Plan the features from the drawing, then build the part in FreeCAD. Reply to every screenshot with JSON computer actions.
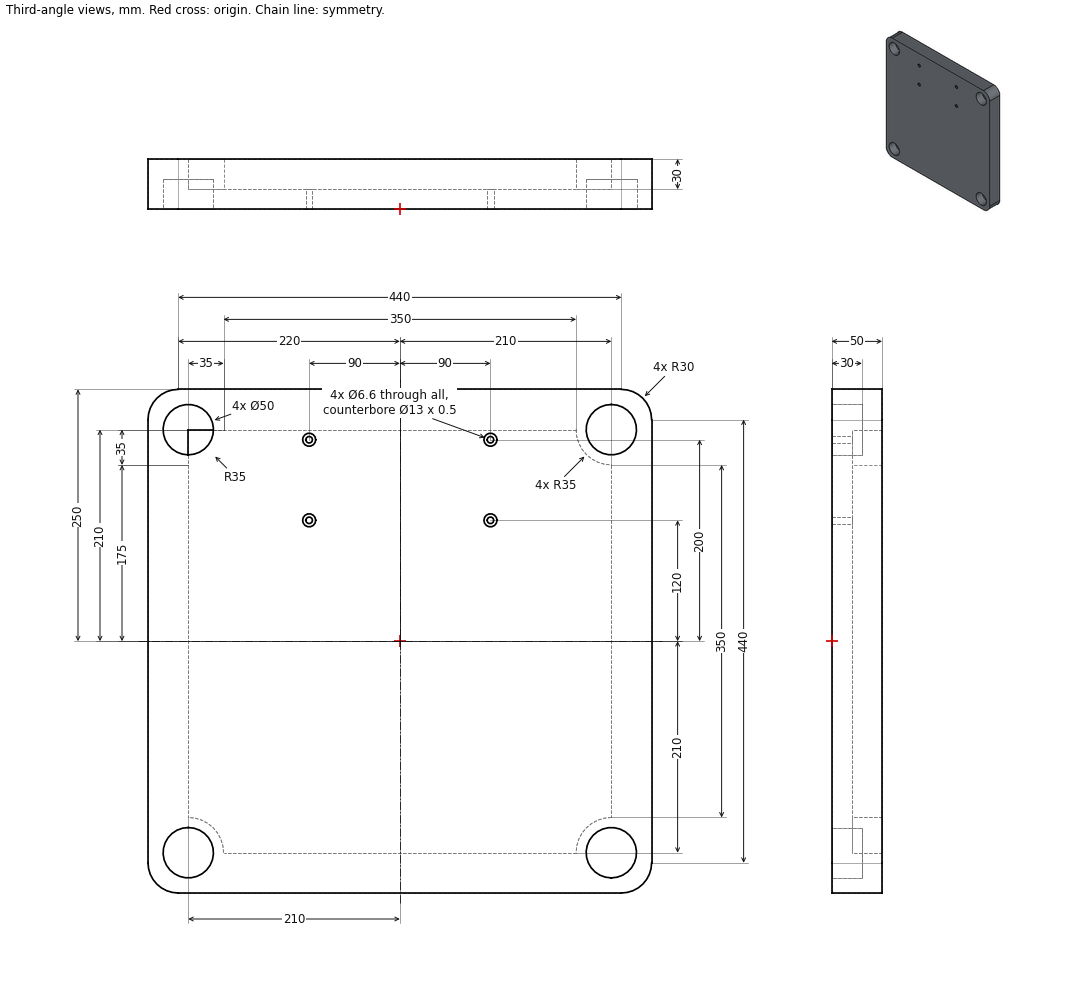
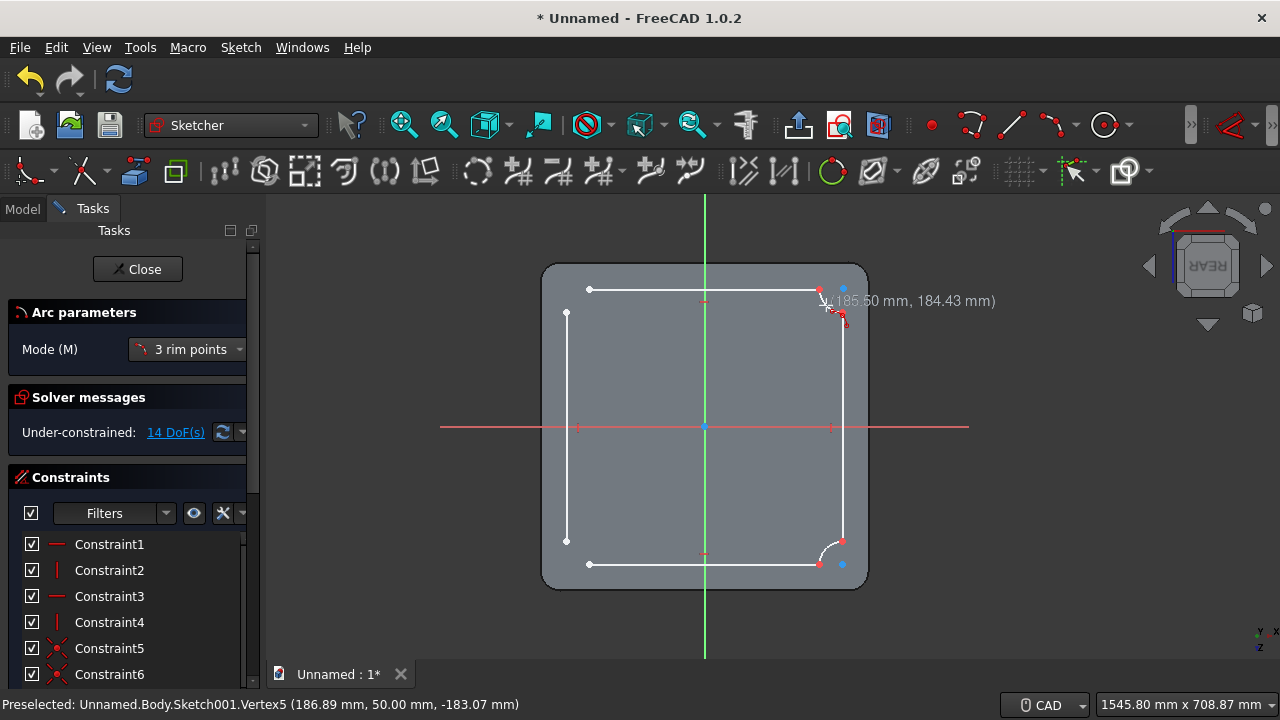
{"action": "left_click", "coordinate": [590, 290]}
{"action": "left_click", "coordinate": [567, 313]}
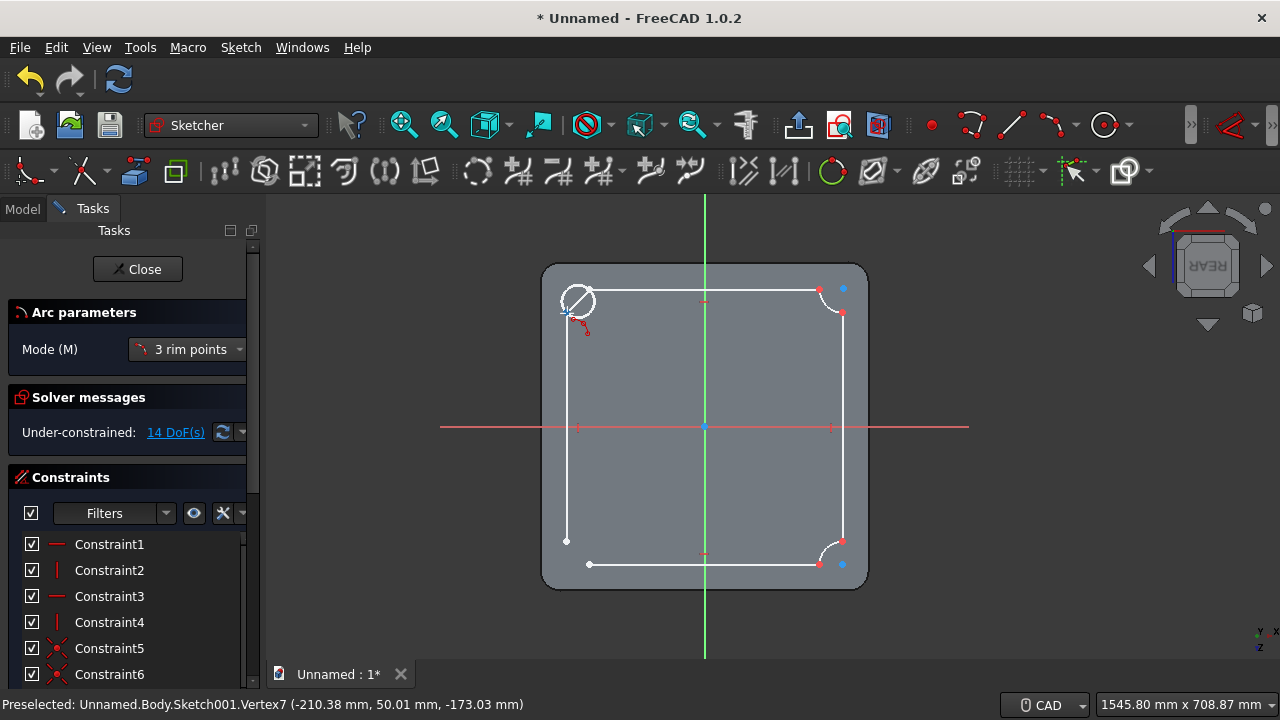
{"action": "scroll", "coordinate": [583, 305], "scroll_direction": "up", "scroll_amount": 5}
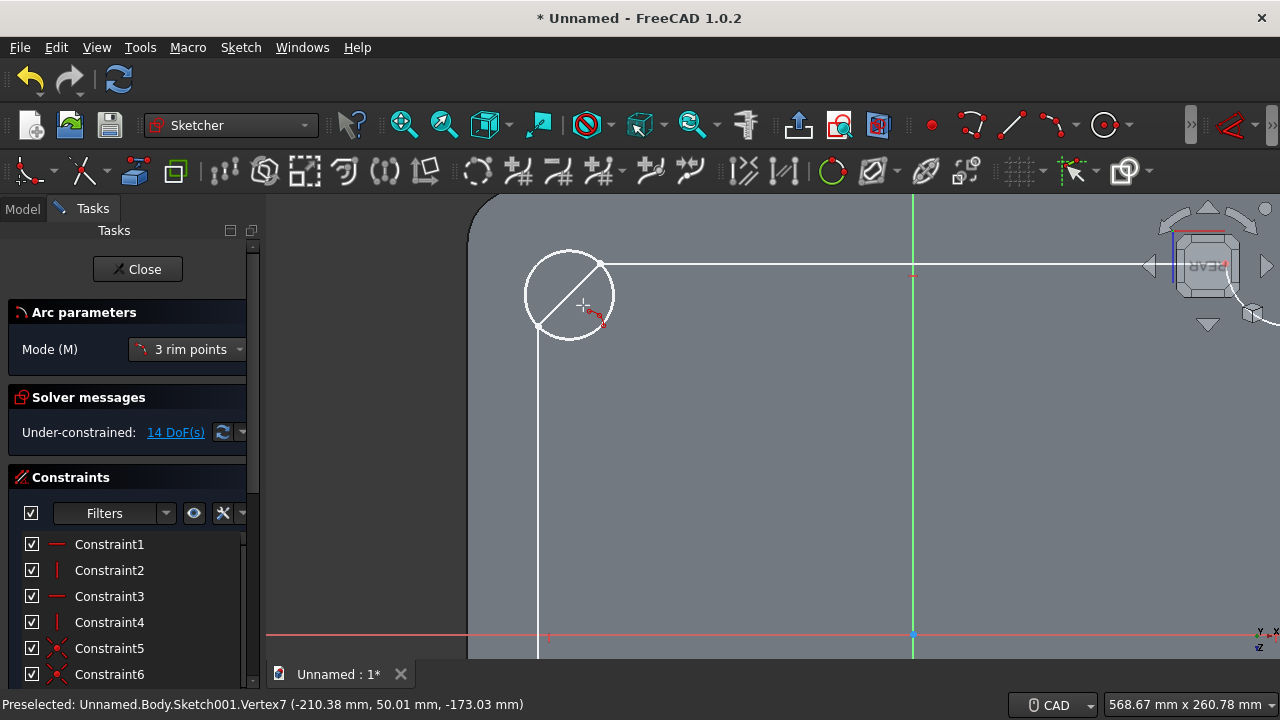
{"action": "left_click", "coordinate": [583, 305]}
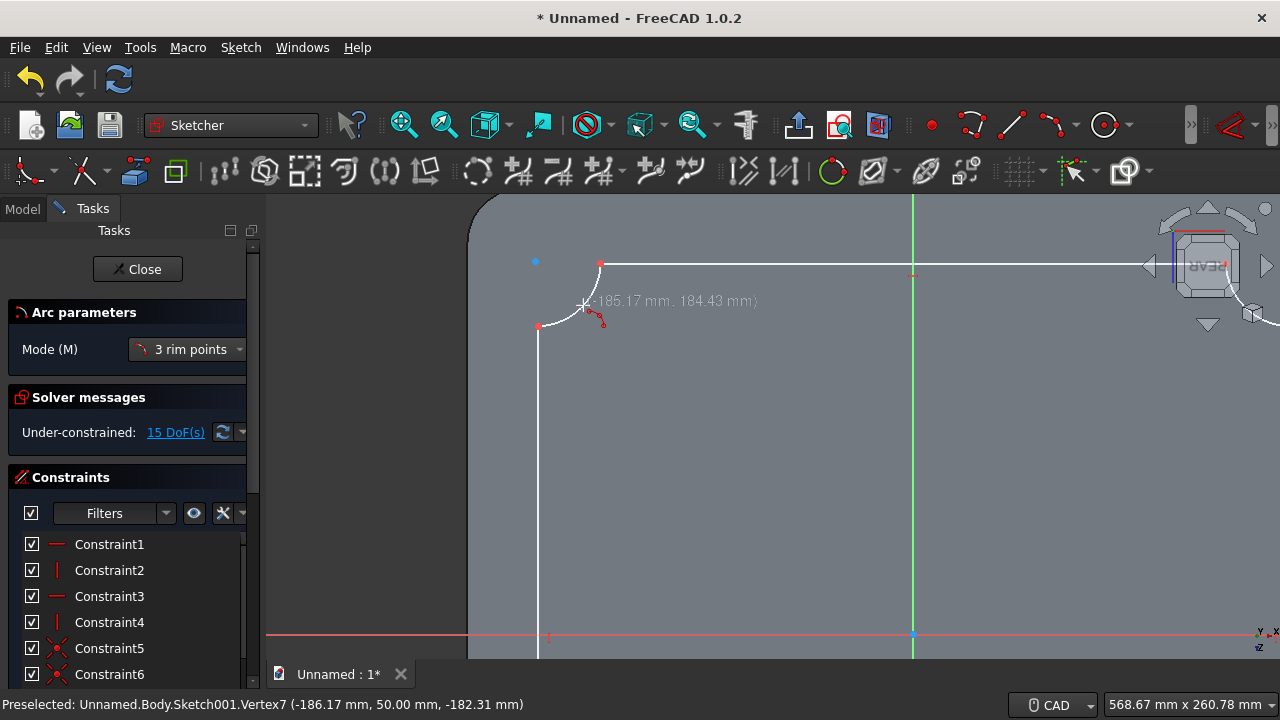
{"action": "scroll", "coordinate": [583, 305], "scroll_direction": "down", "scroll_amount": 5}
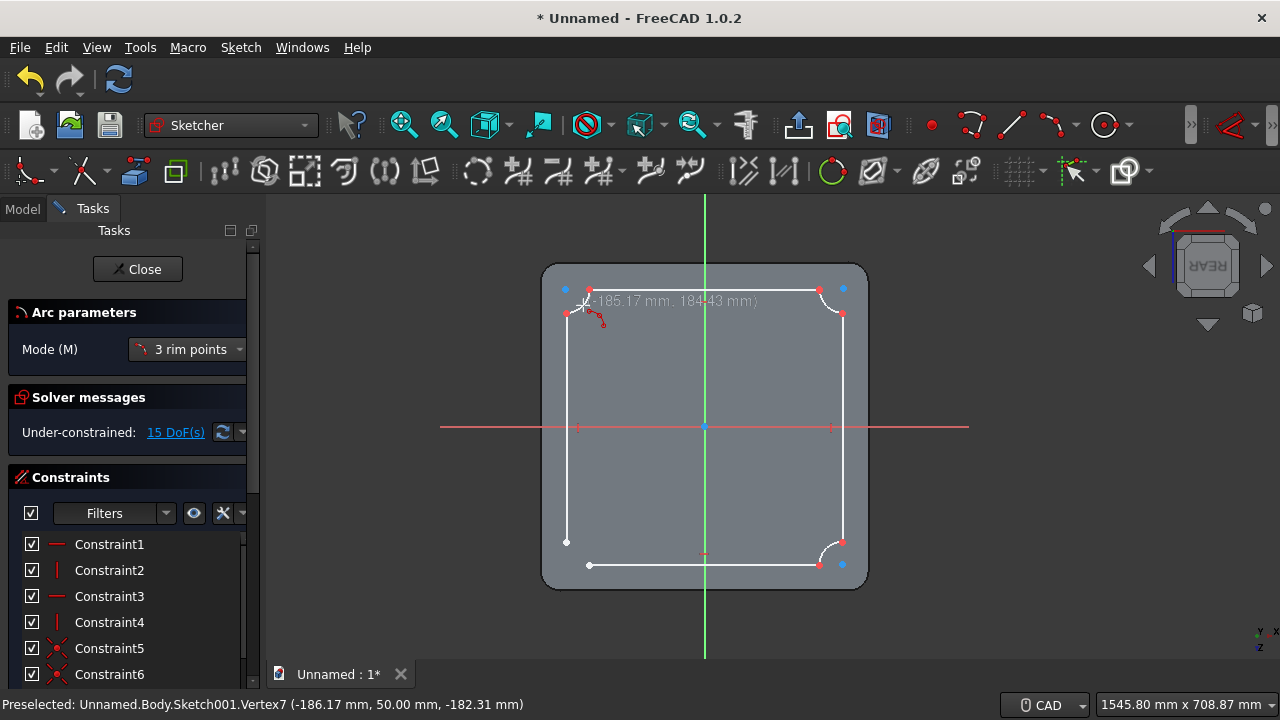
{"action": "left_click", "coordinate": [567, 542]}
{"action": "left_click", "coordinate": [590, 565]}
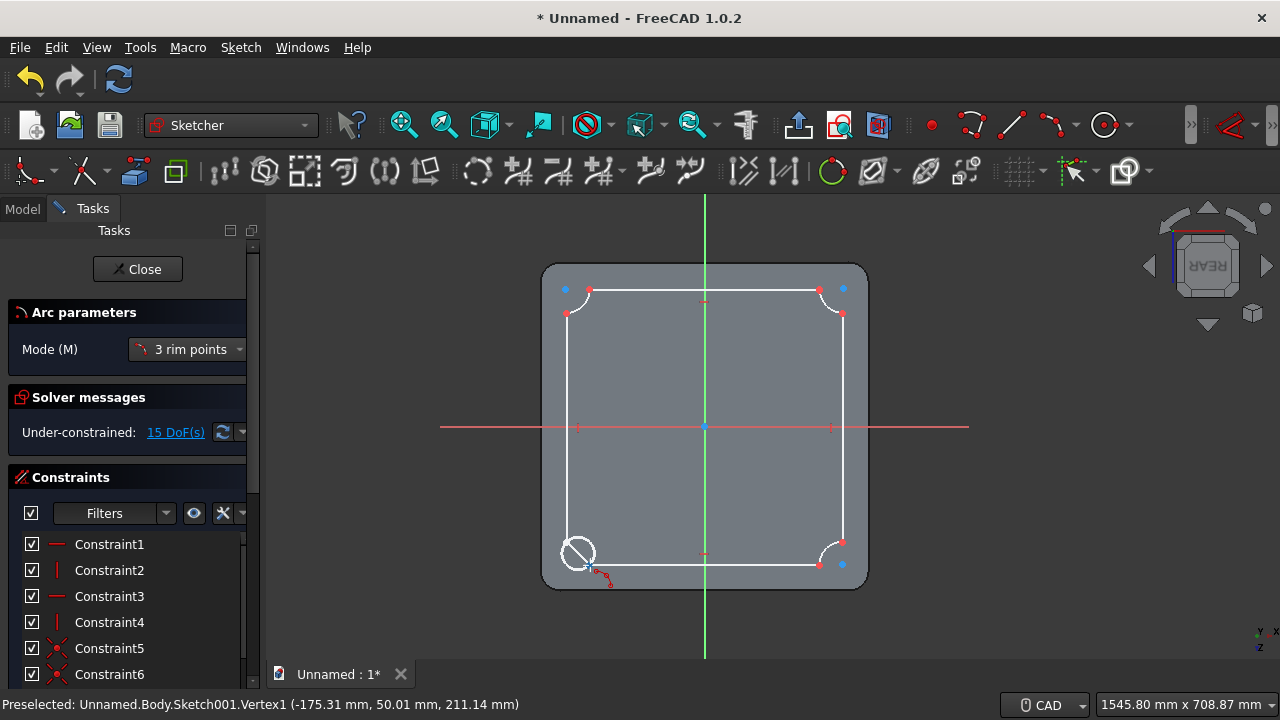
{"action": "scroll", "coordinate": [583, 548], "scroll_direction": "up", "scroll_amount": 5}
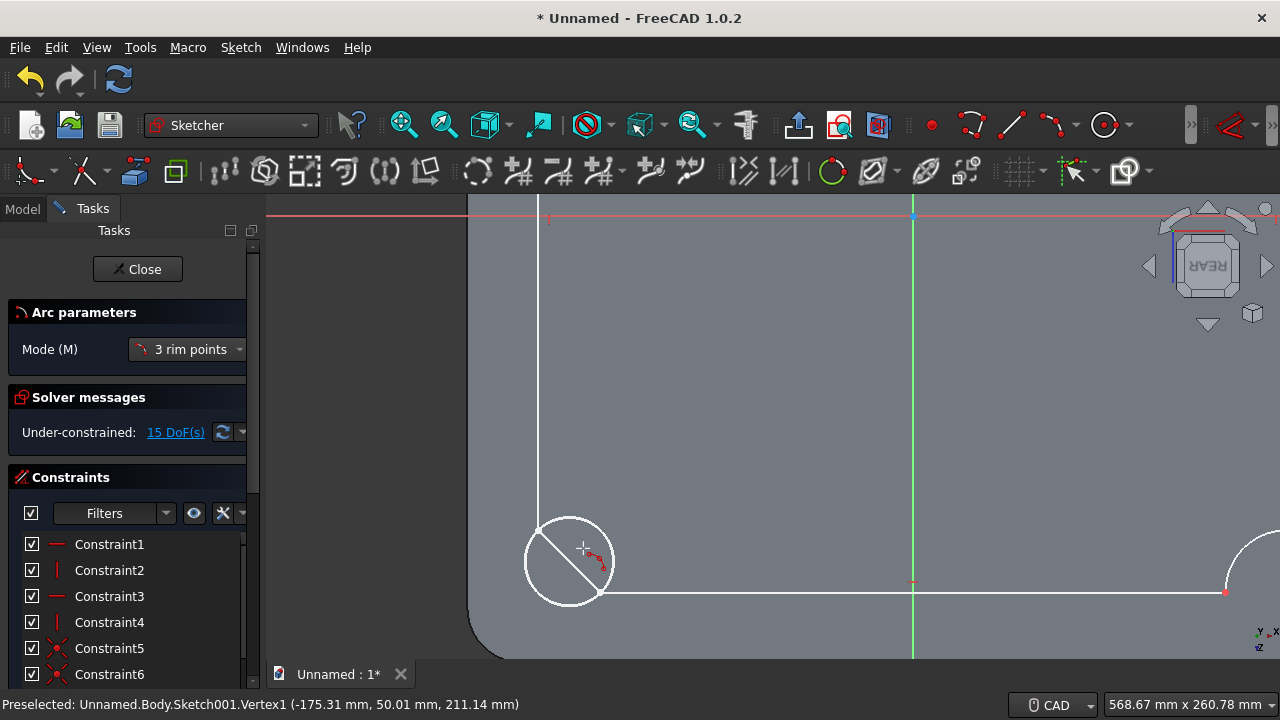
{"action": "left_click", "coordinate": [583, 547]}
{"action": "key", "text": "Escape"}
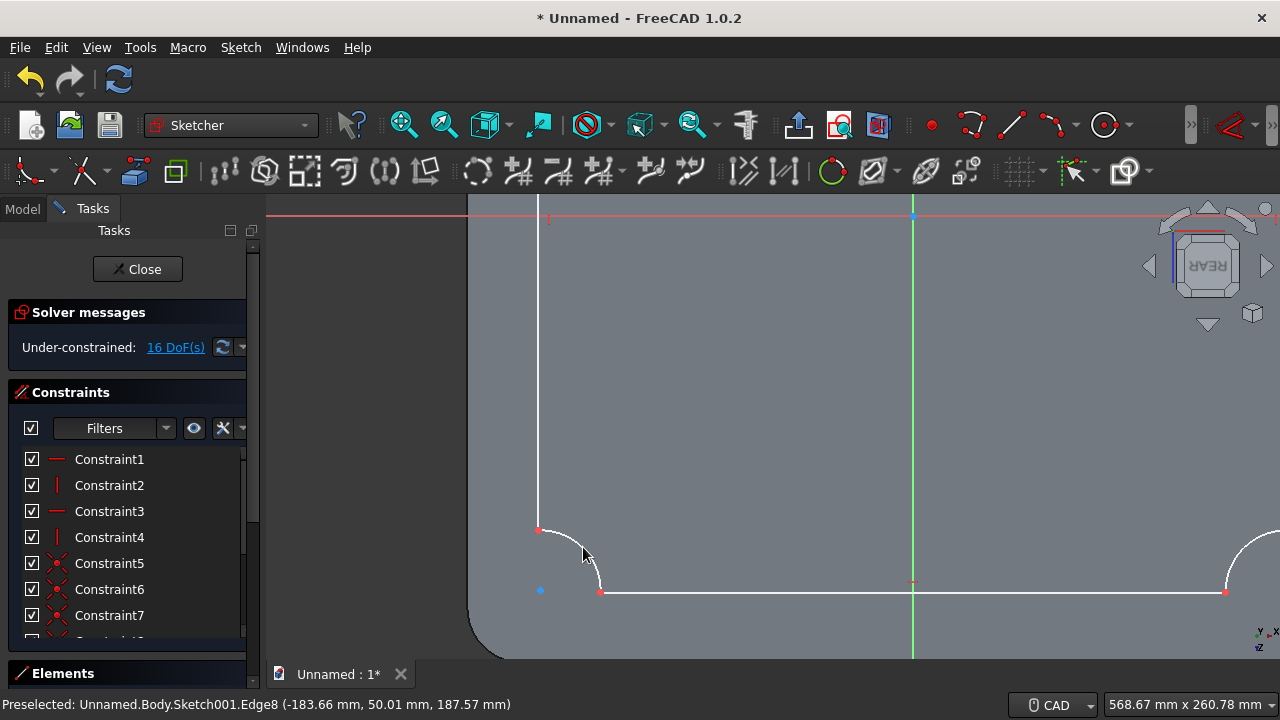
{"action": "scroll", "coordinate": [583, 549], "scroll_direction": "down", "scroll_amount": 5}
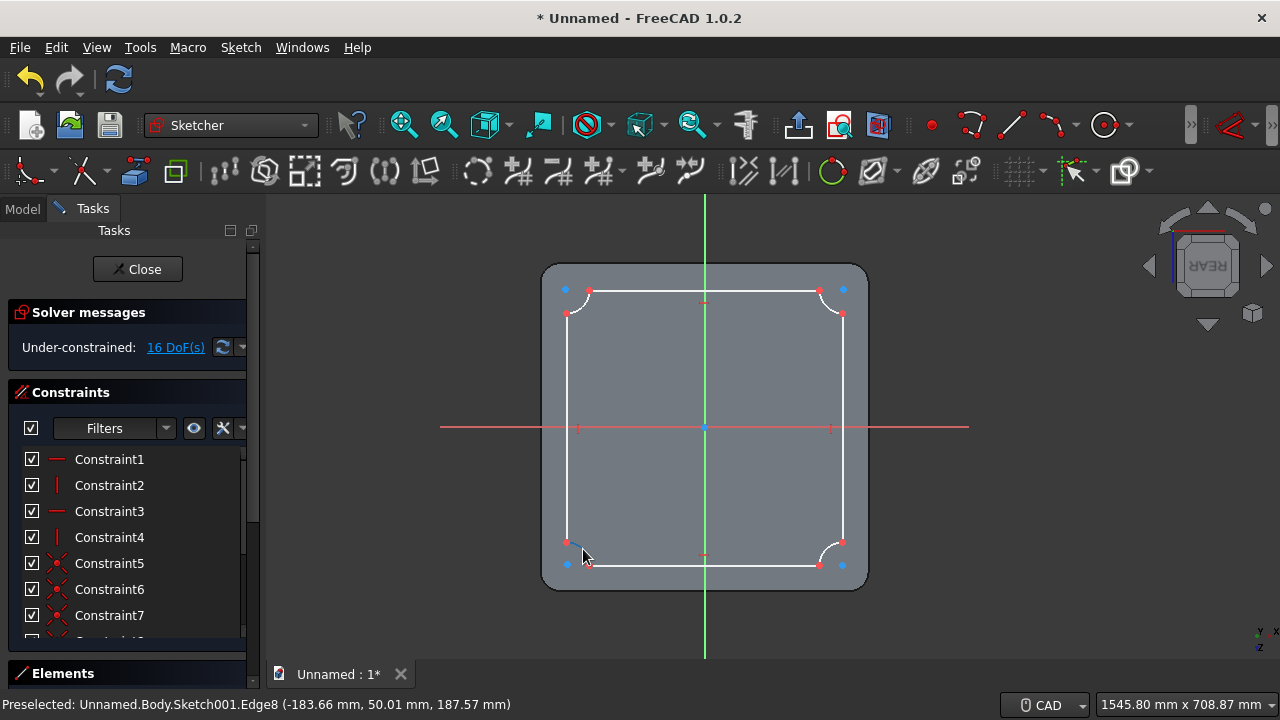
{"action": "scroll", "coordinate": [832, 545], "scroll_direction": "up", "scroll_amount": 2}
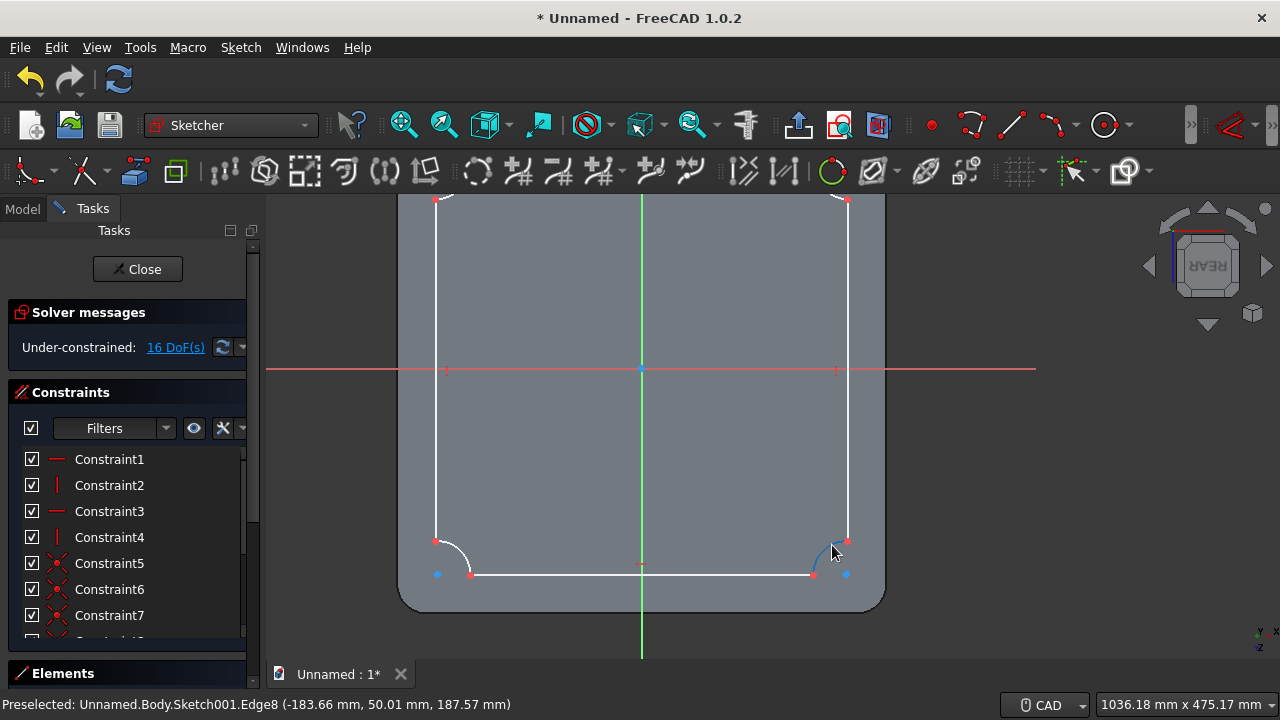
{"action": "left_click", "coordinate": [832, 545]}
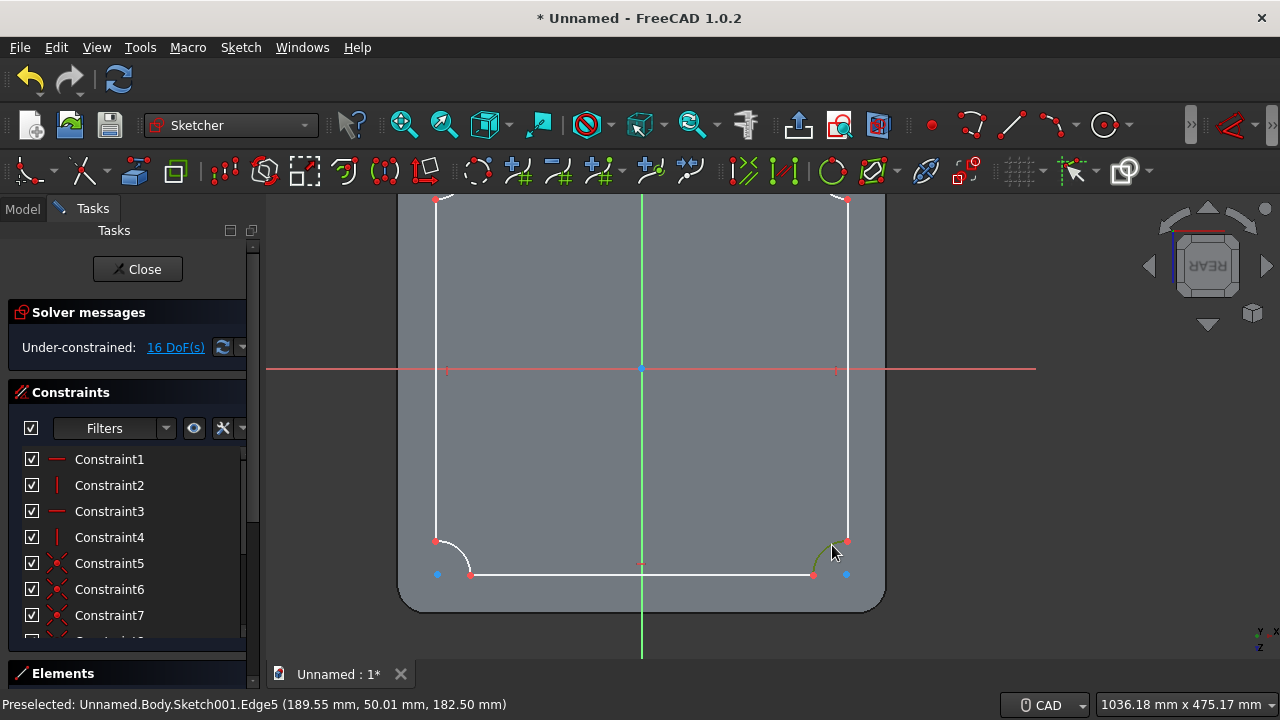
{"action": "scroll", "coordinate": [832, 544], "scroll_direction": "down", "scroll_amount": 2}